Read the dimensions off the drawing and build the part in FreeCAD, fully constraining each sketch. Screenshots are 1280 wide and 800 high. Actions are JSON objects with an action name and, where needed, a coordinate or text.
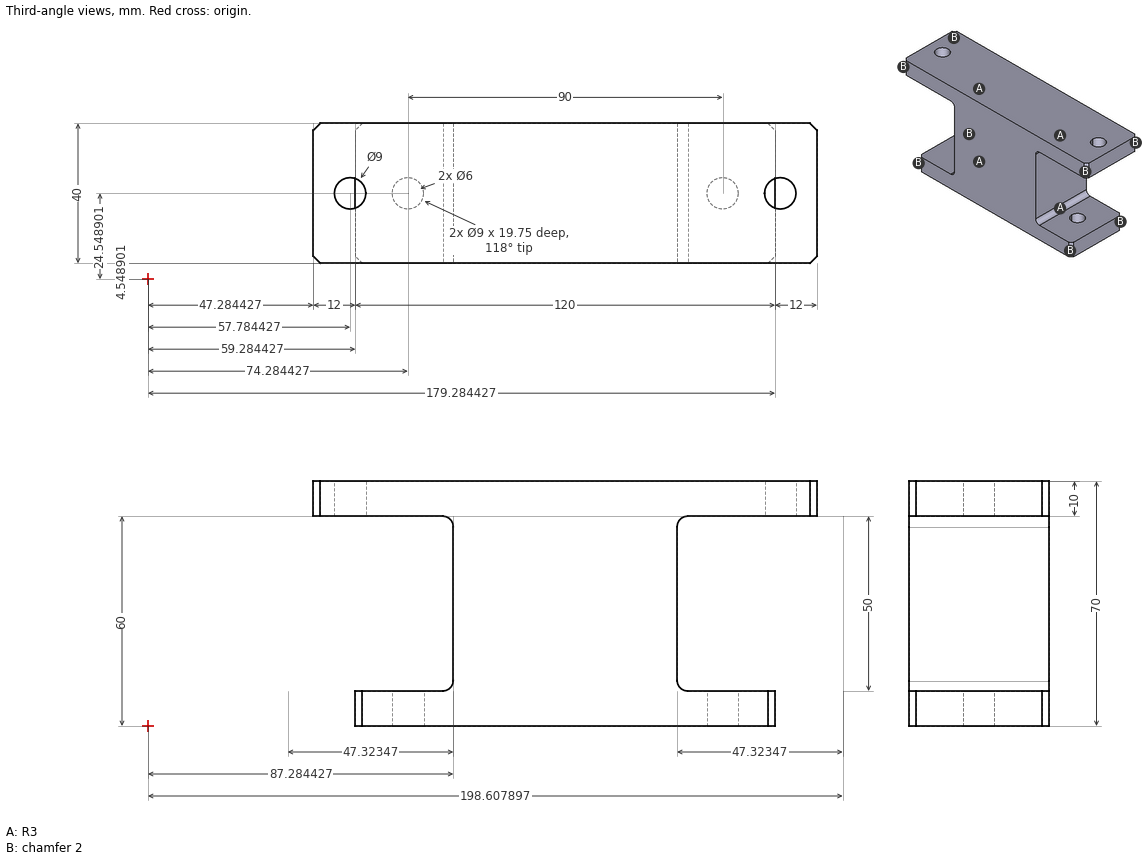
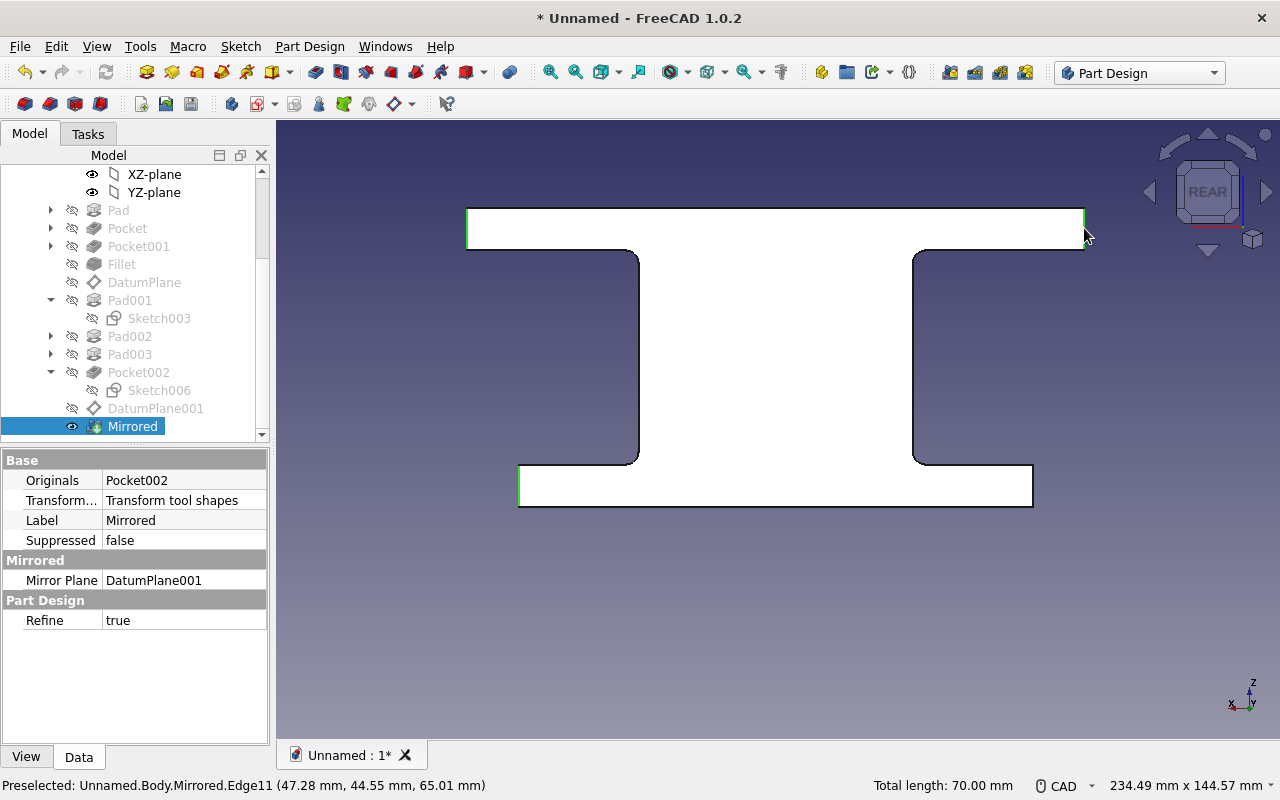
{"action": "left_click", "coordinate": [1033, 485], "text": "ctrl"}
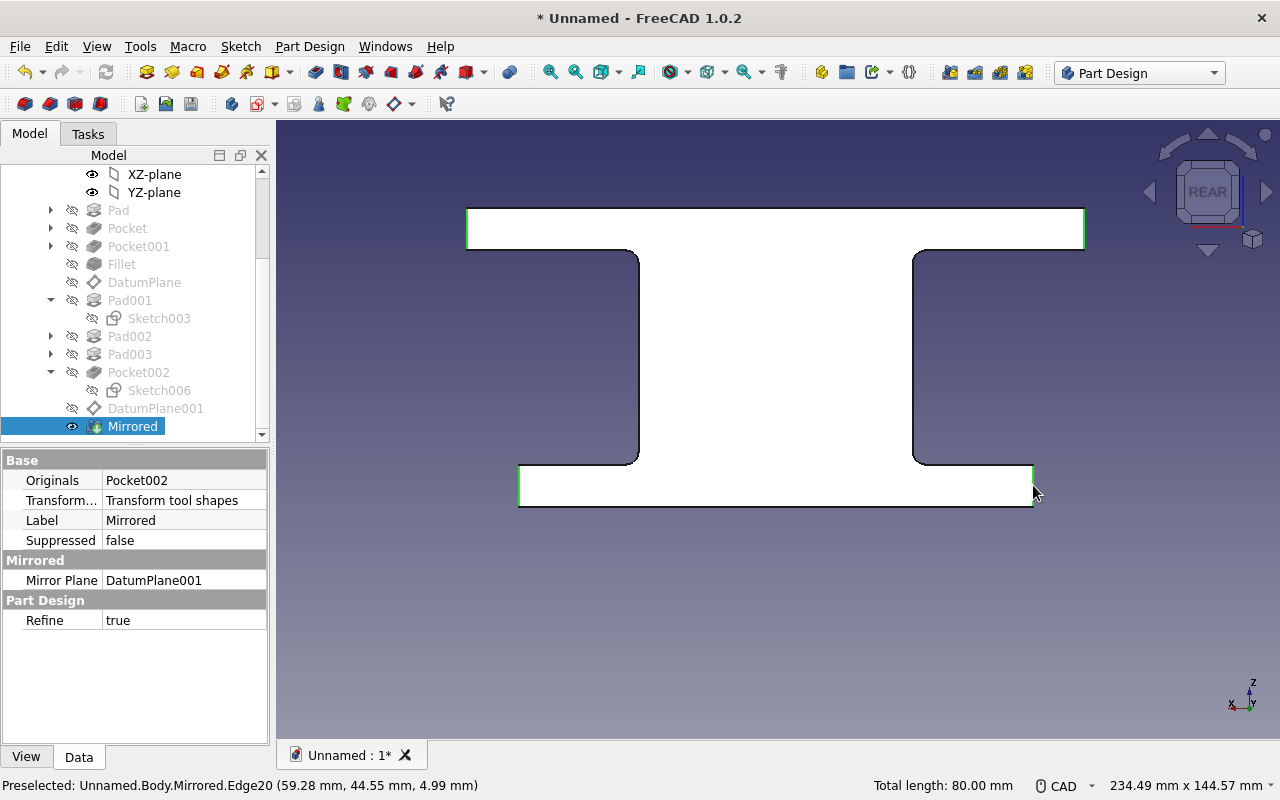
{"action": "left_click", "coordinate": [50, 104]}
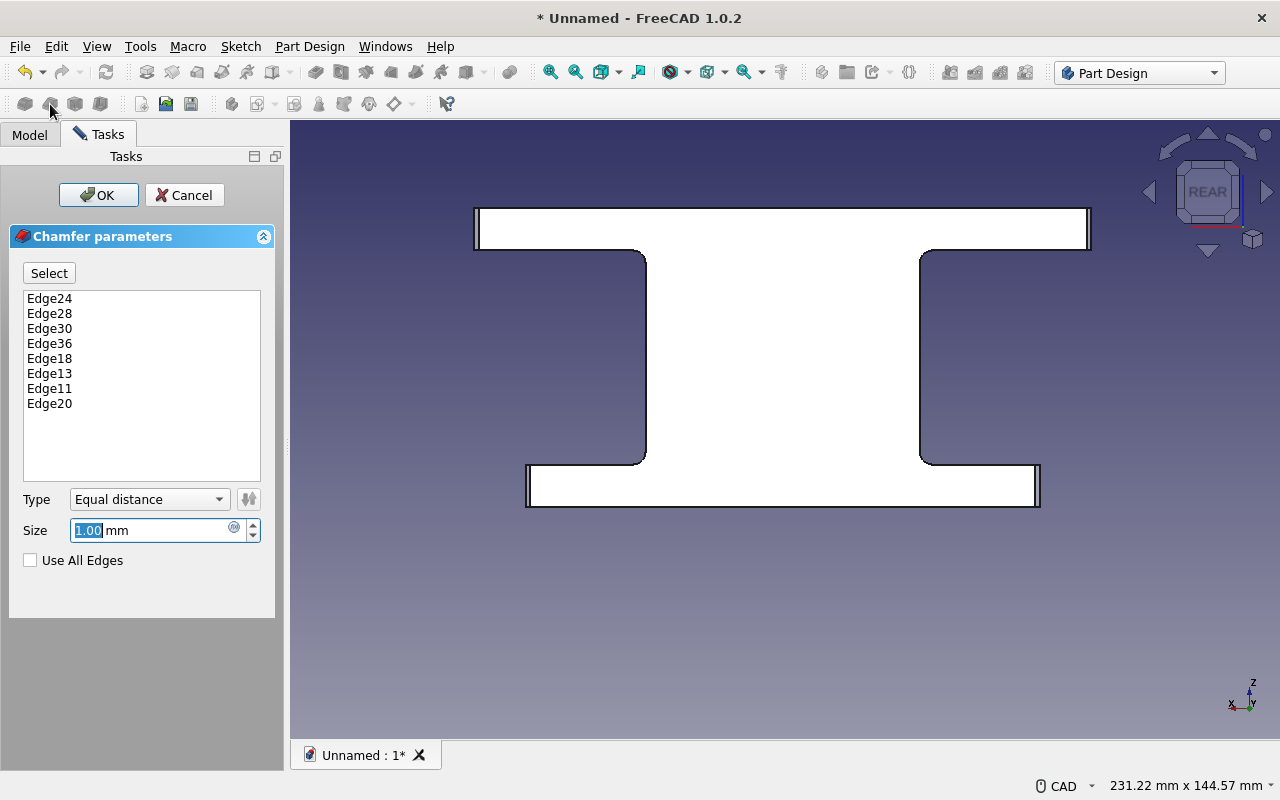
{"action": "type", "text": "2"}
{"action": "key", "text": "Tab"}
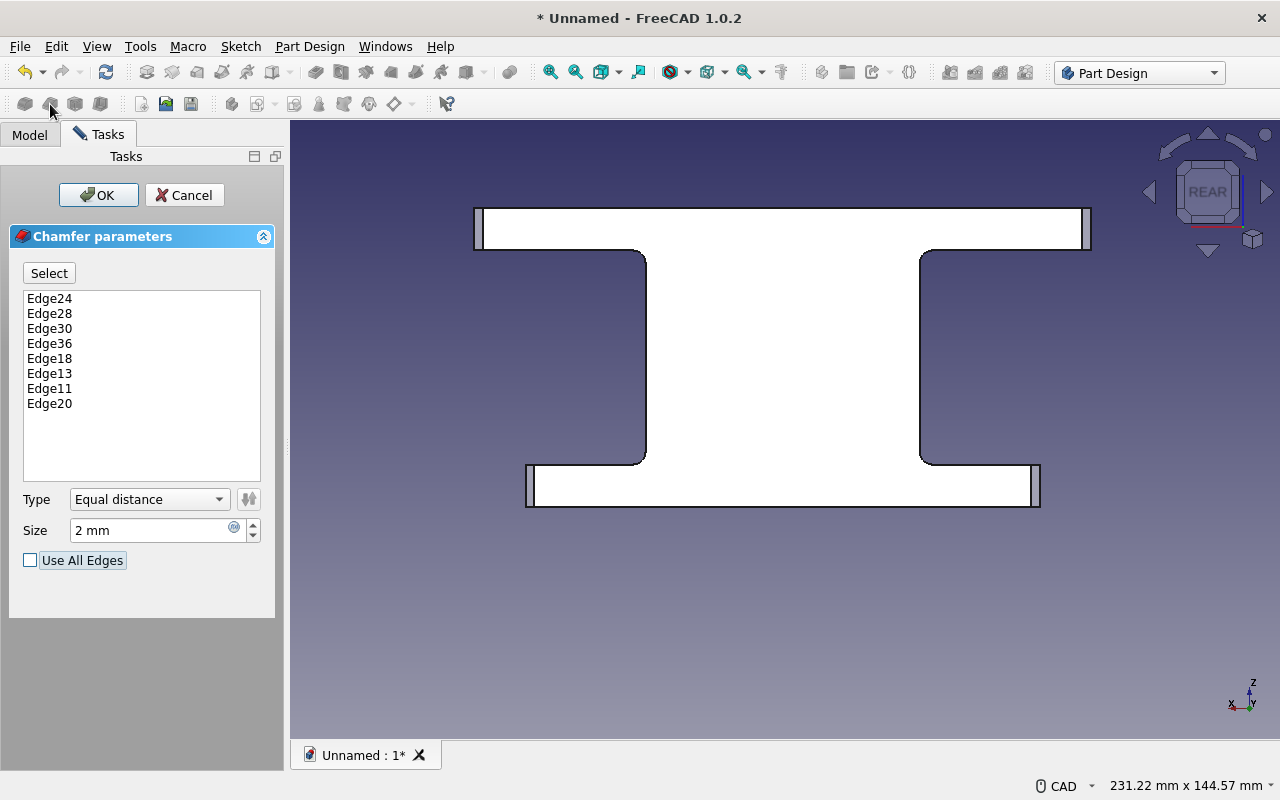
{"action": "left_click", "coordinate": [99, 195]}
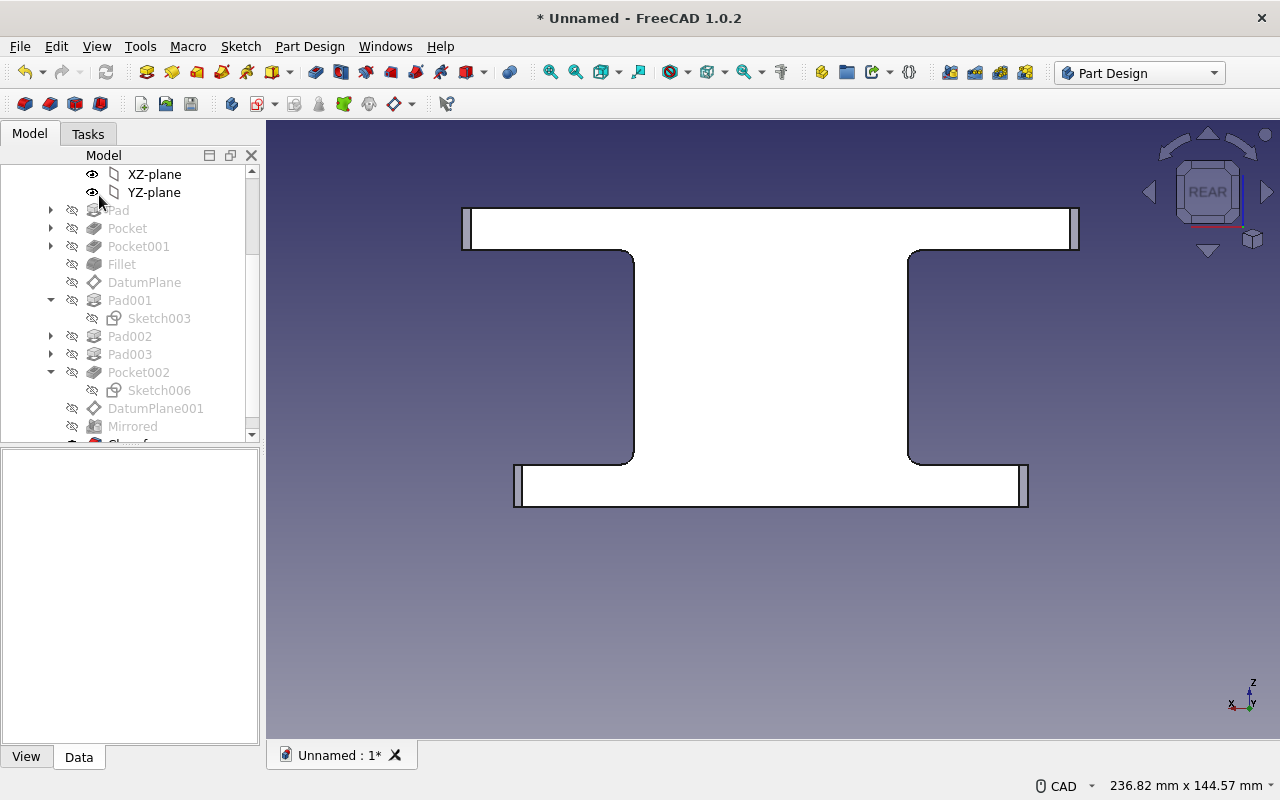
{"action": "key", "text": "5"}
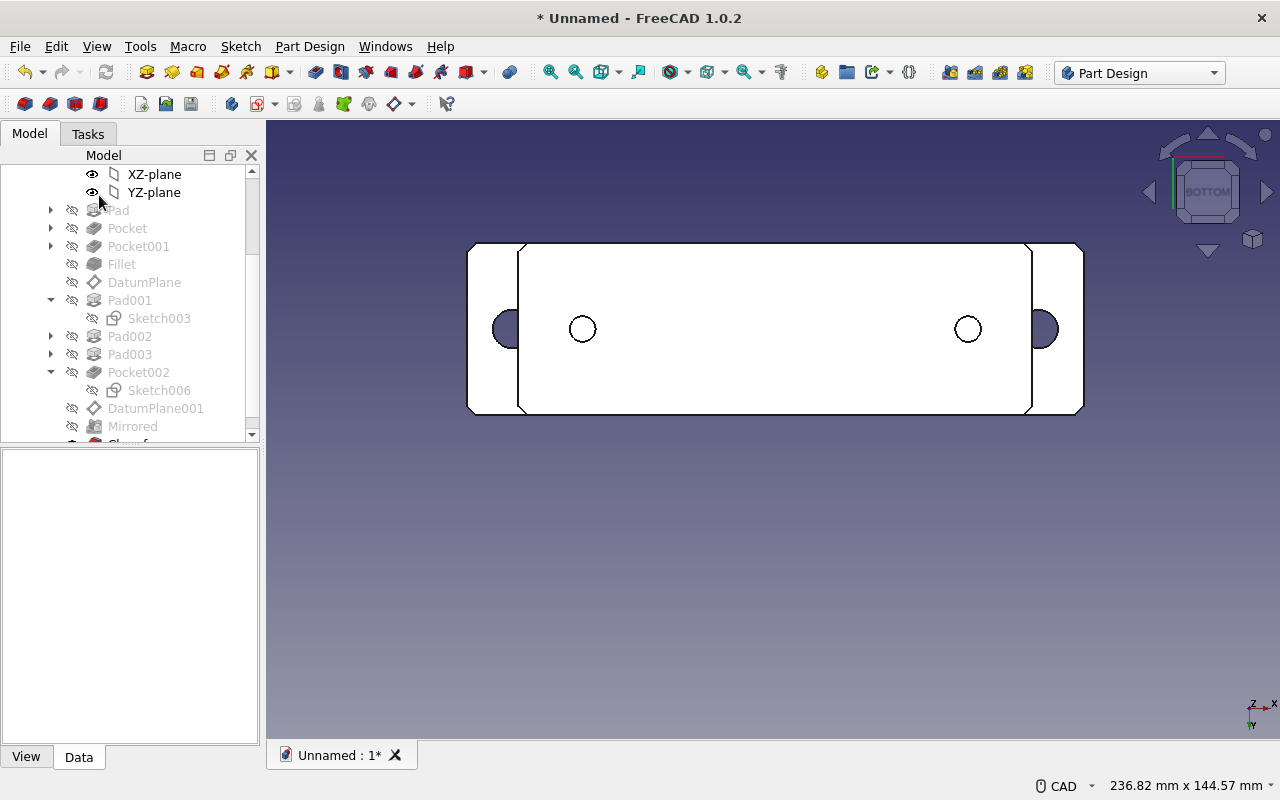
{"action": "left_click", "coordinate": [849, 328]}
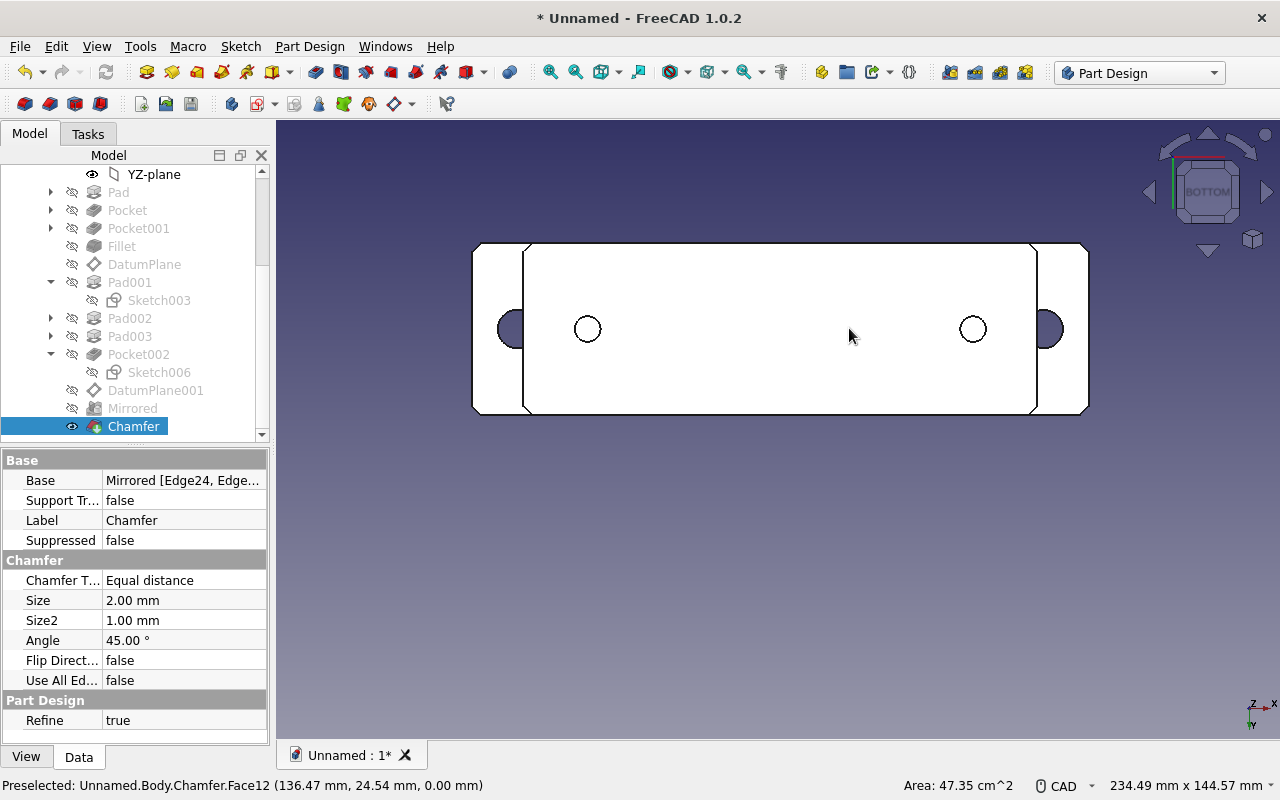
{"action": "left_click", "coordinate": [256, 104]}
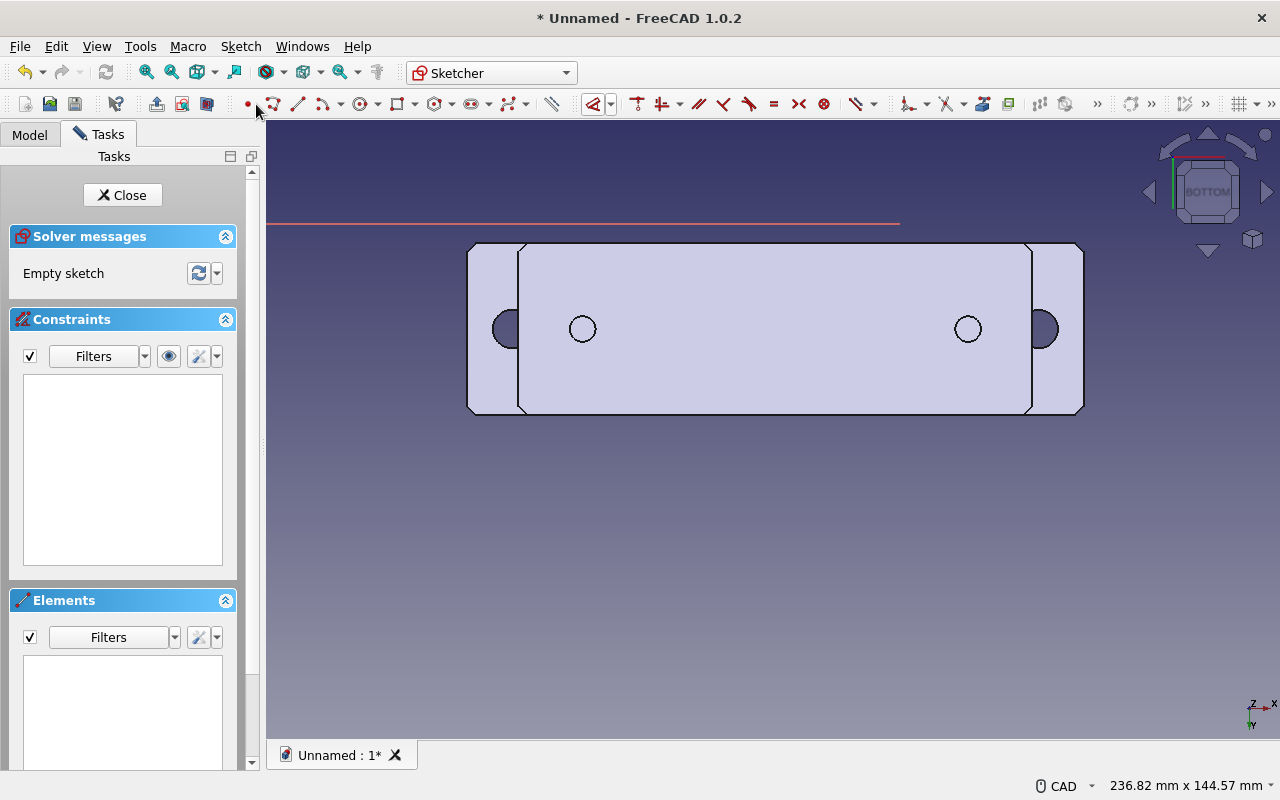
{"action": "scroll", "coordinate": [1059, 711], "scroll_direction": "down", "scroll_amount": 1}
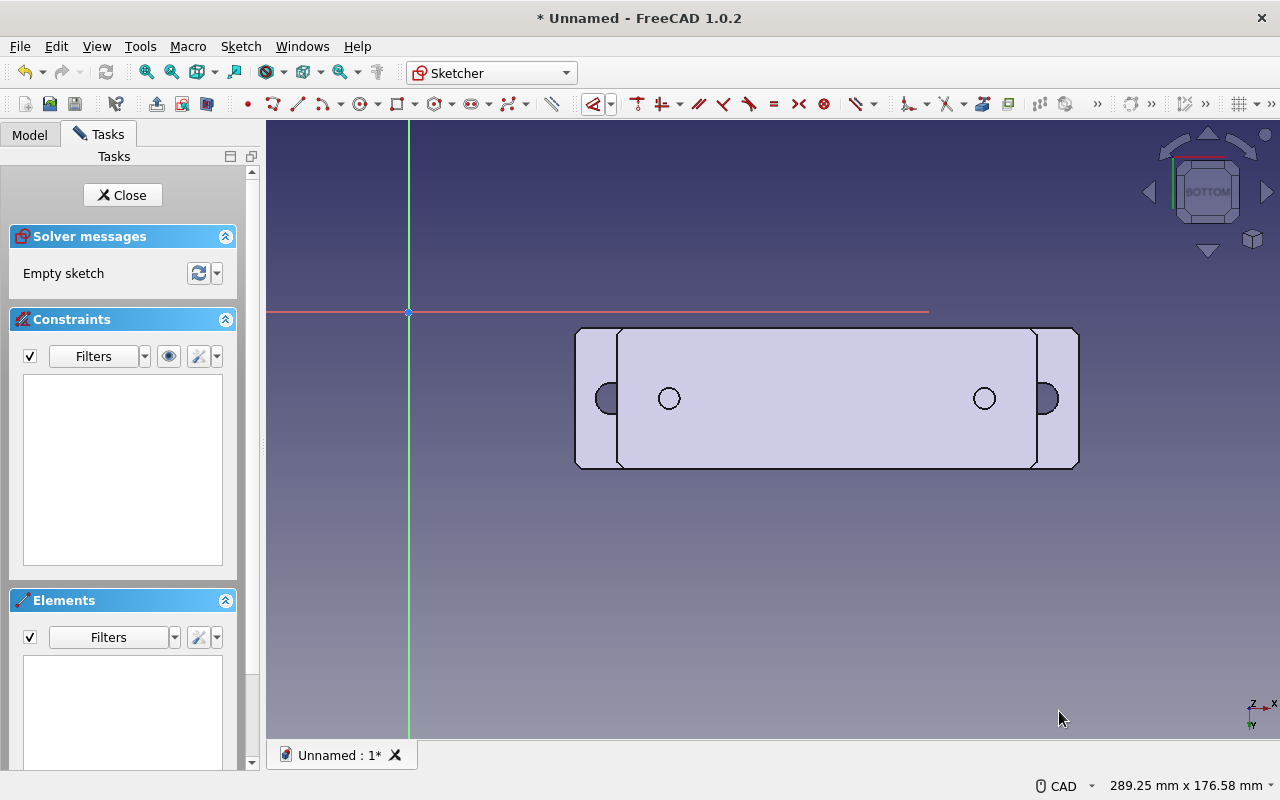
{"action": "key", "text": "g c"}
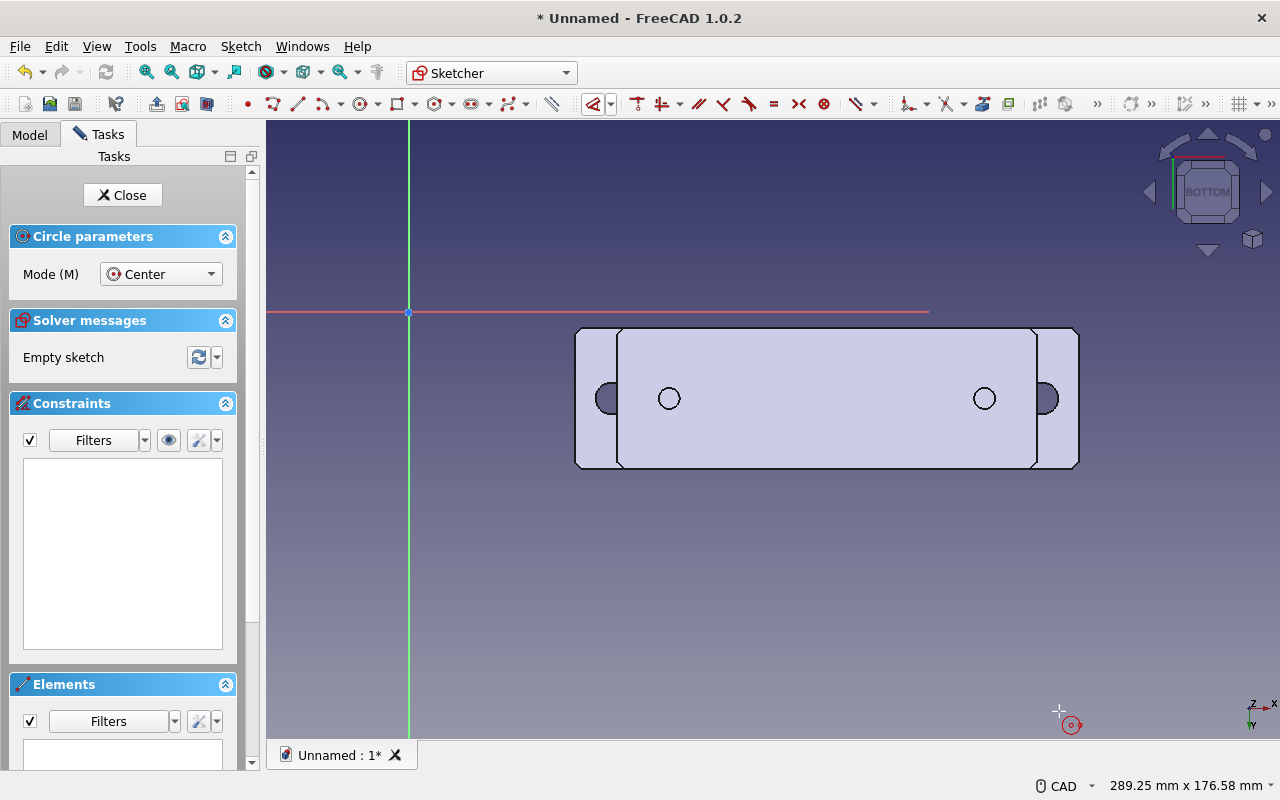
{"action": "scroll", "coordinate": [669, 398], "scroll_direction": "up", "scroll_amount": 2}